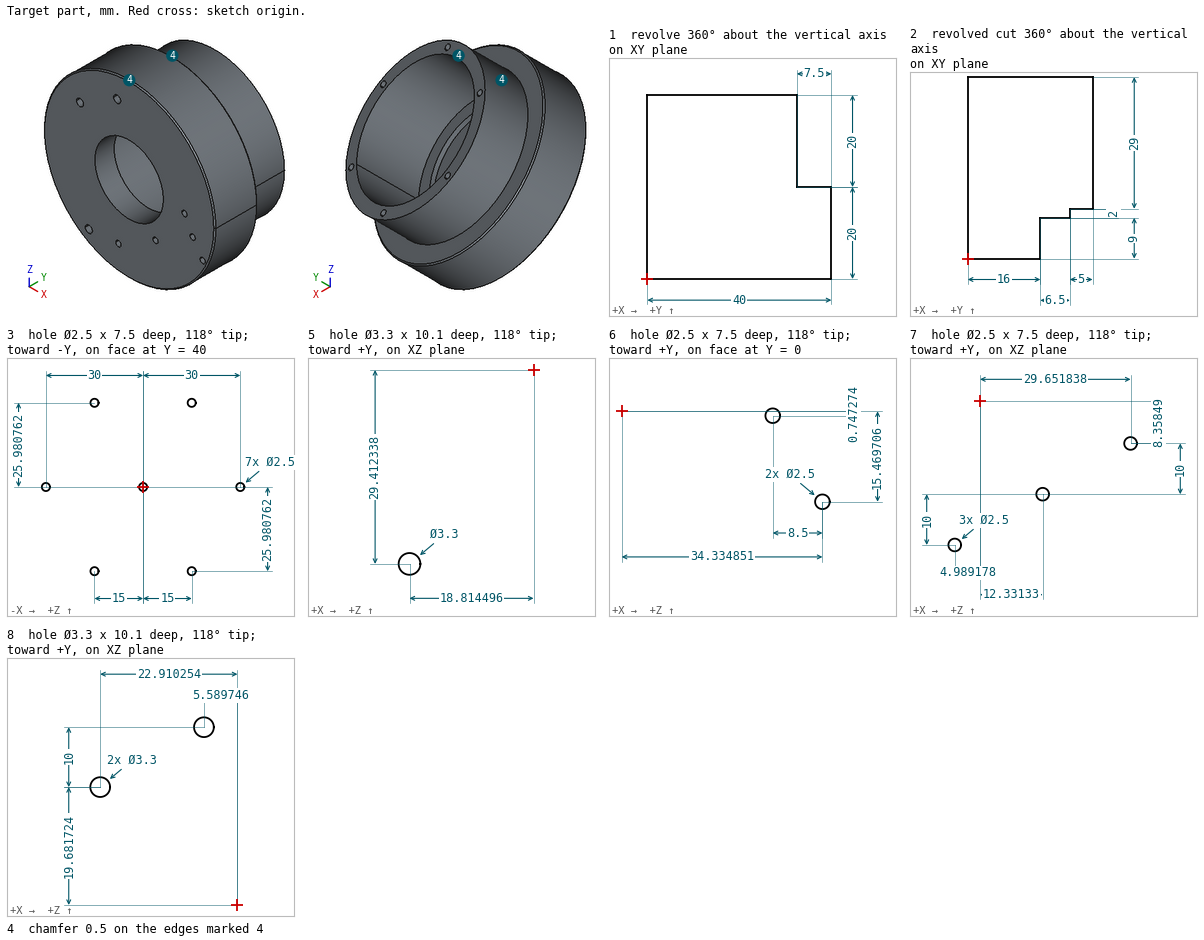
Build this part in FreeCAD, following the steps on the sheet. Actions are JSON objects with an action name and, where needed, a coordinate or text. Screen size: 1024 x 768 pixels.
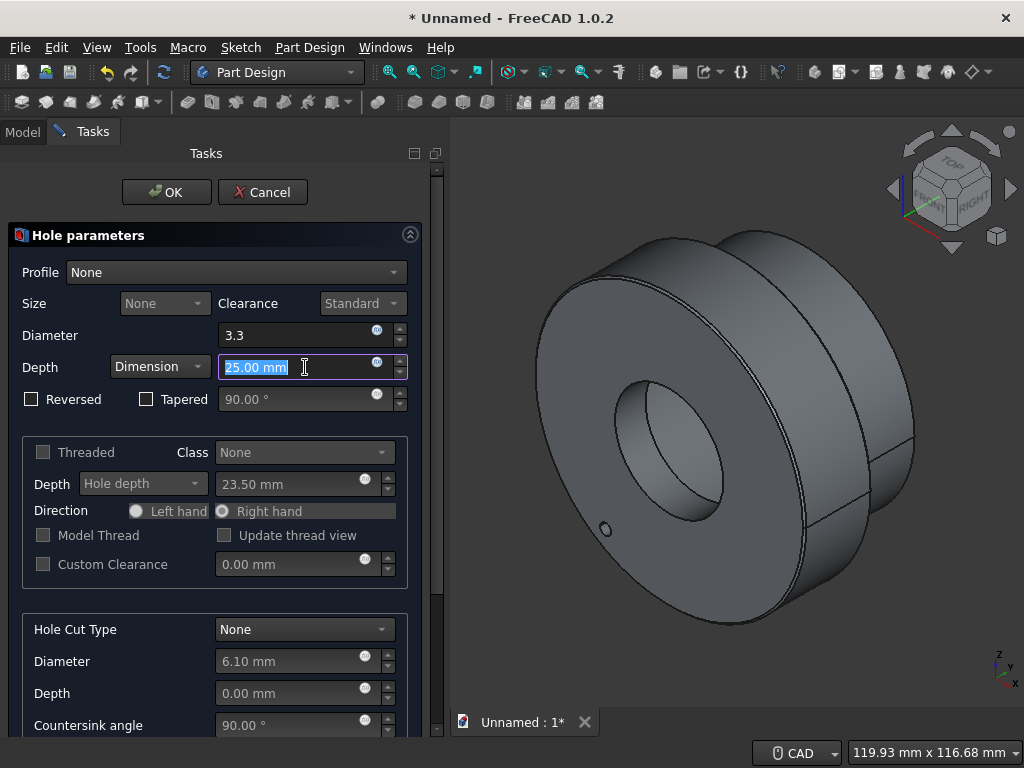
{"action": "type", "text": "10.1"}
{"action": "key", "text": "Tab"}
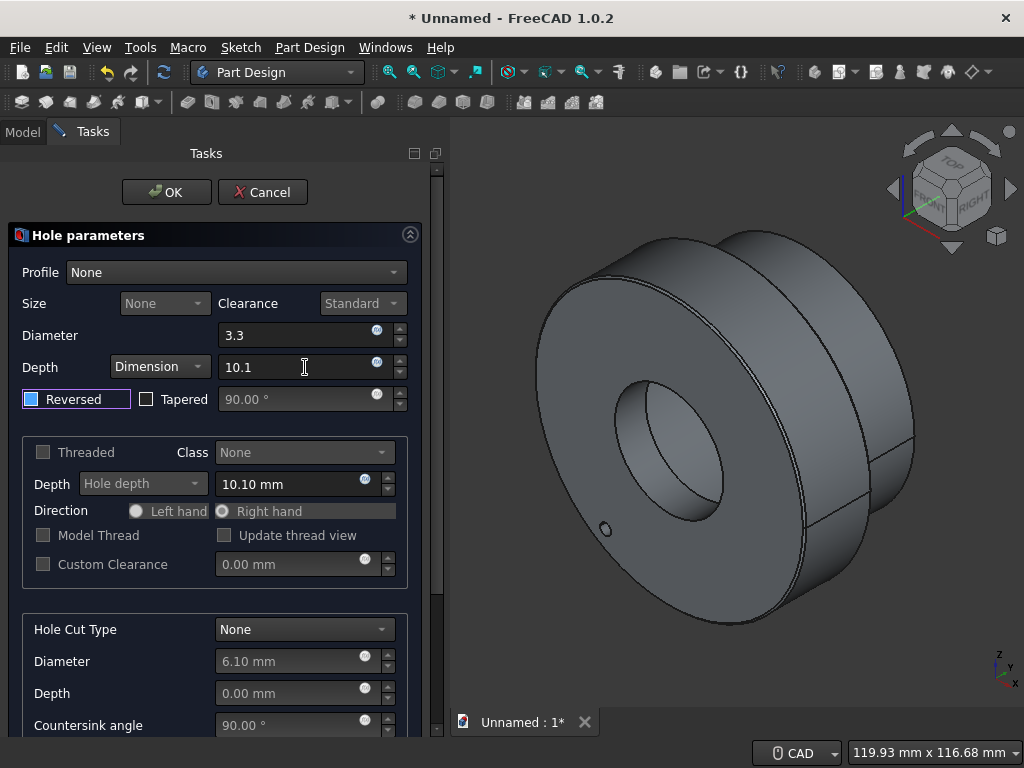
{"action": "left_click", "coordinate": [167, 192]}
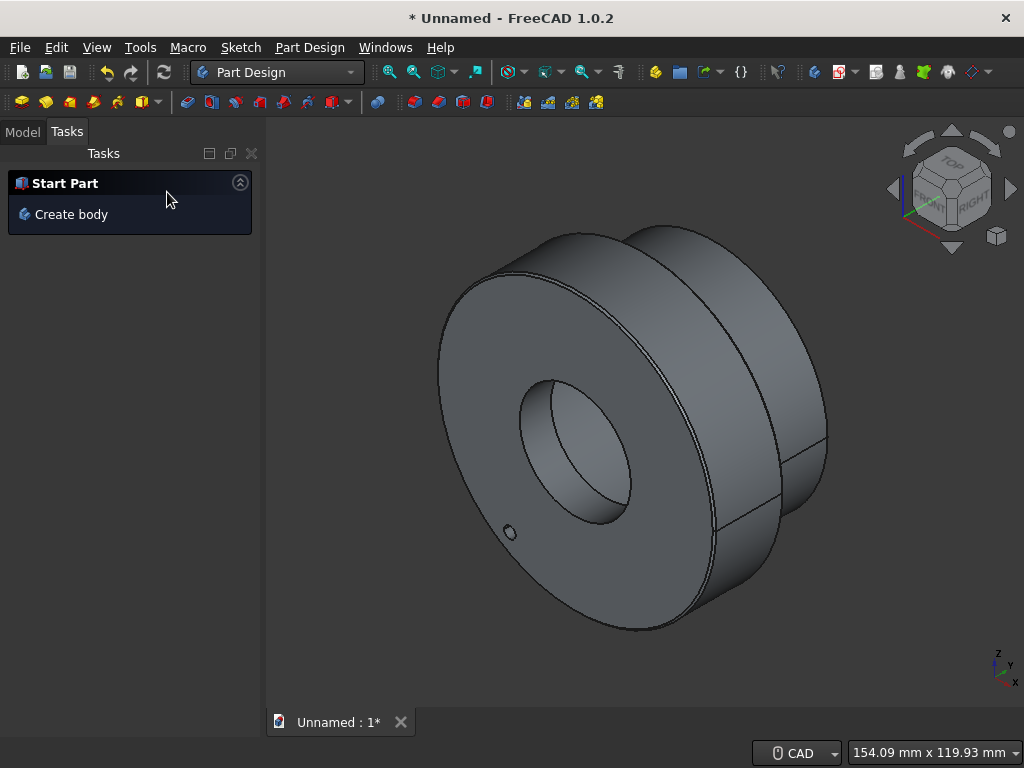
{"action": "left_click", "coordinate": [654, 451]}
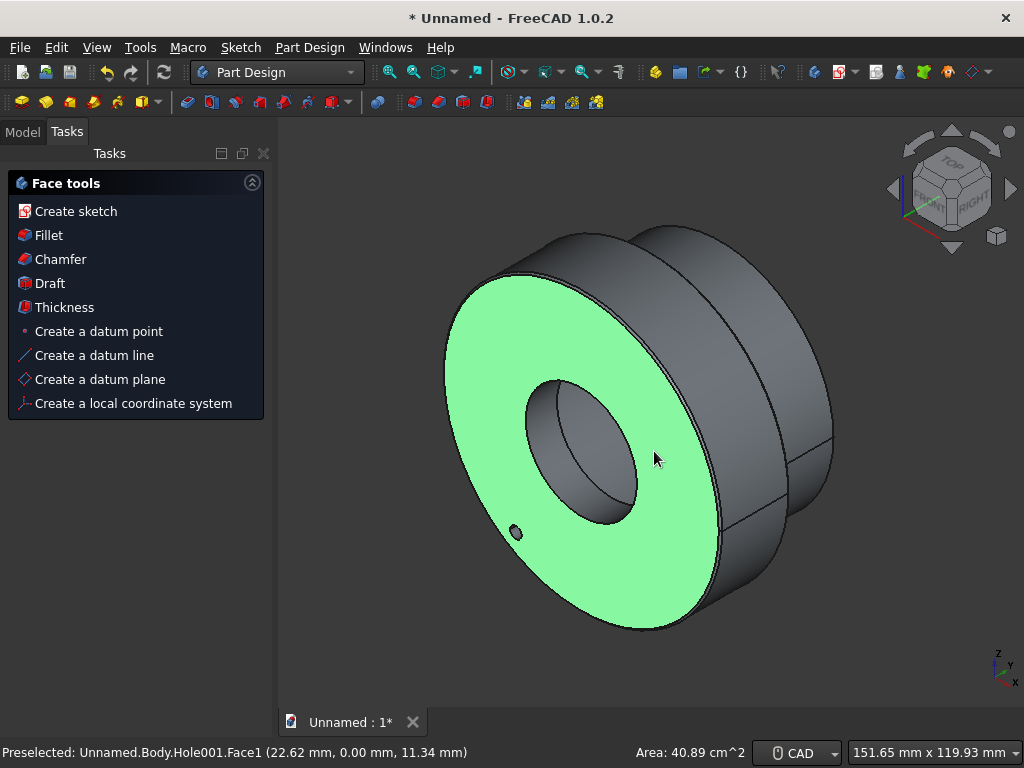
{"action": "left_click", "coordinate": [840, 72]}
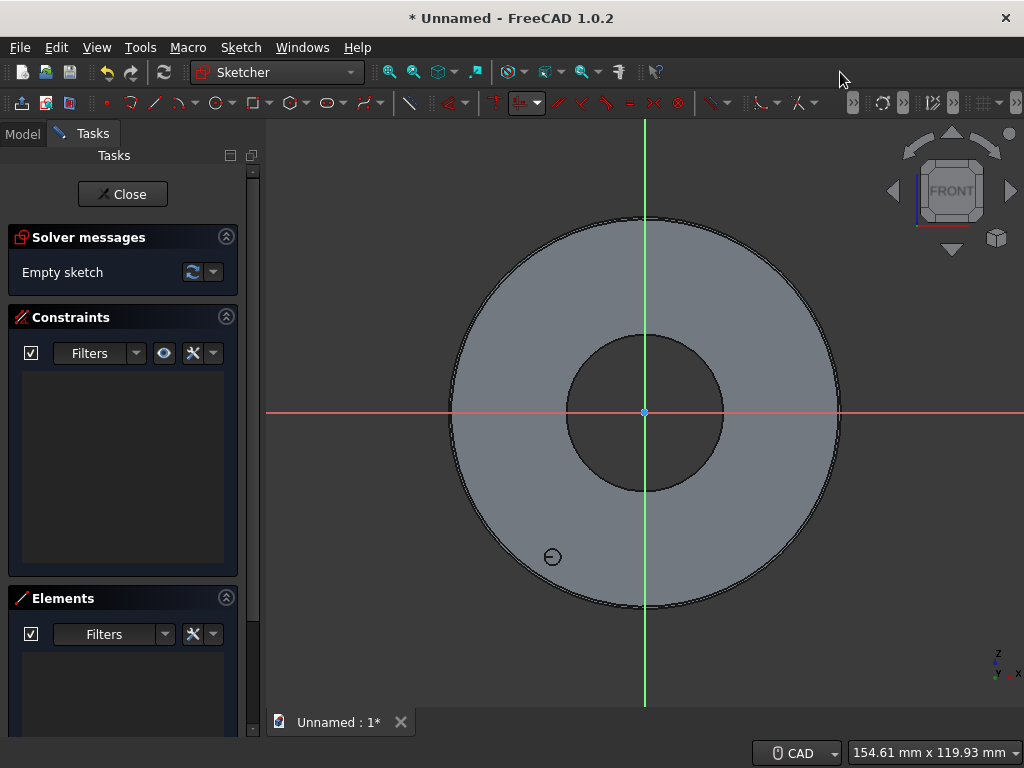
{"action": "scroll", "coordinate": [859, 485], "scroll_direction": "up", "scroll_amount": 4}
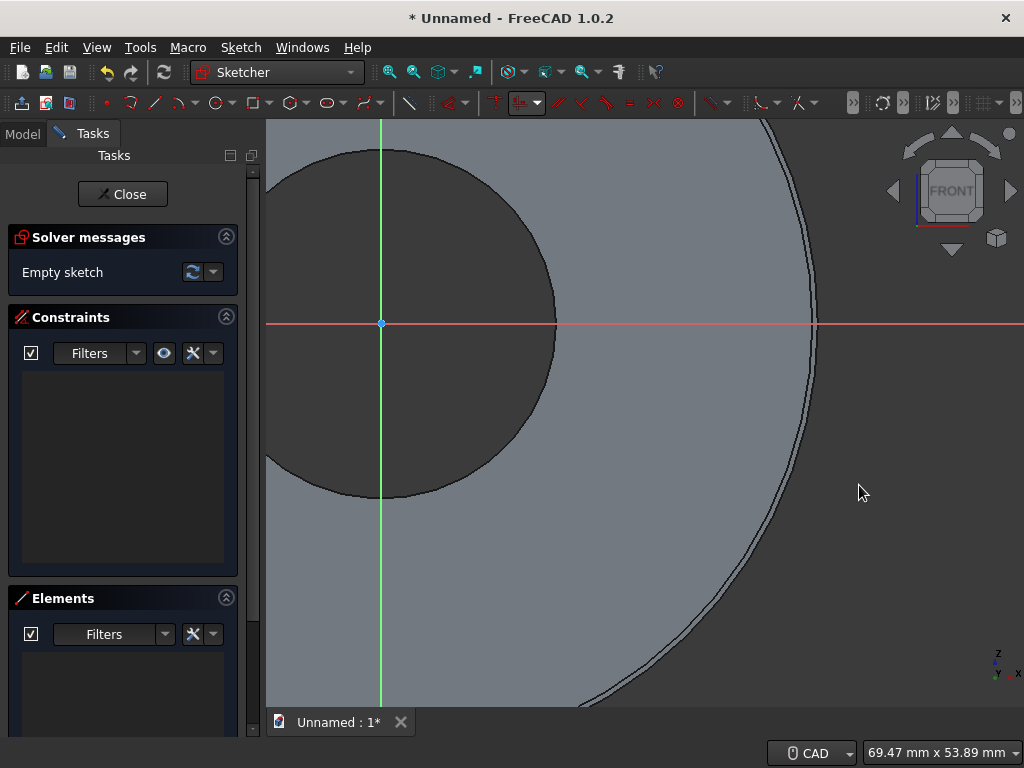
{"action": "left_click", "coordinate": [216, 104]}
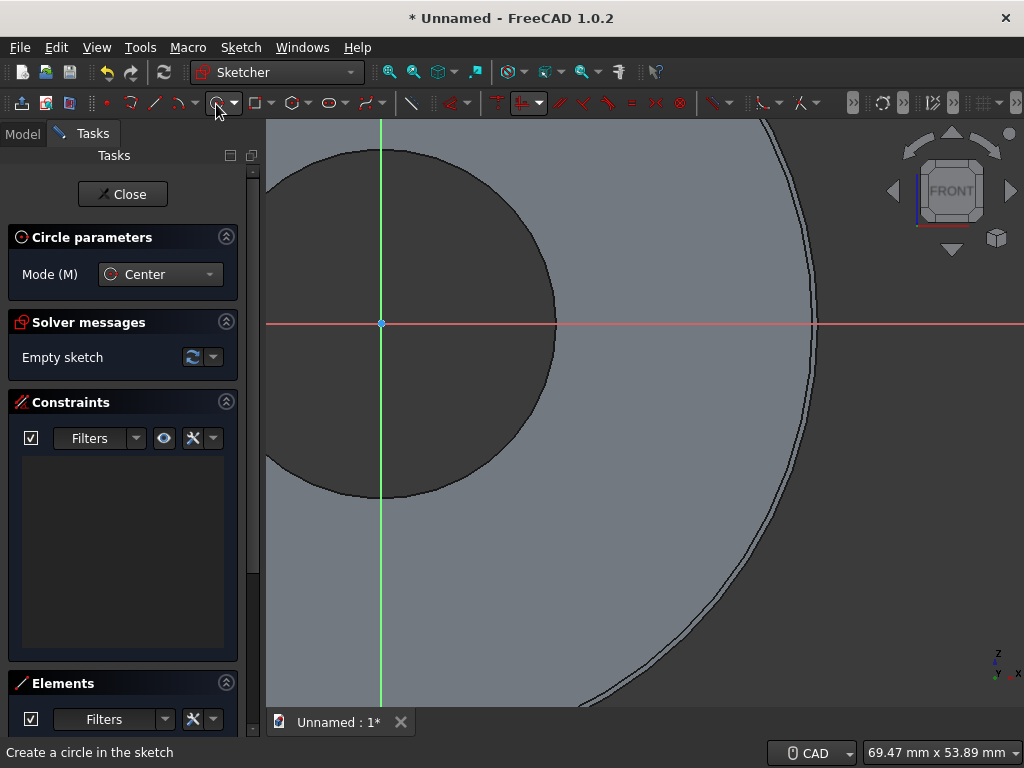
{"action": "scroll", "coordinate": [756, 493], "scroll_direction": "up", "scroll_amount": 3}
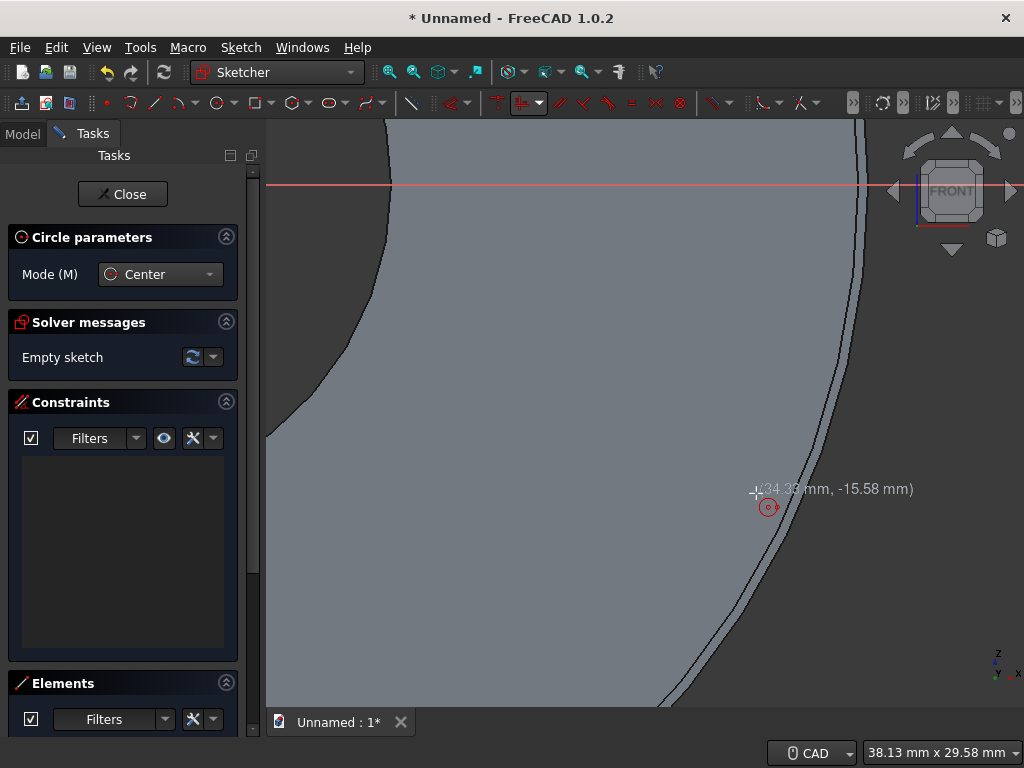
{"action": "left_click", "coordinate": [756, 492]}
{"action": "mouse_move", "coordinate": [773, 475]}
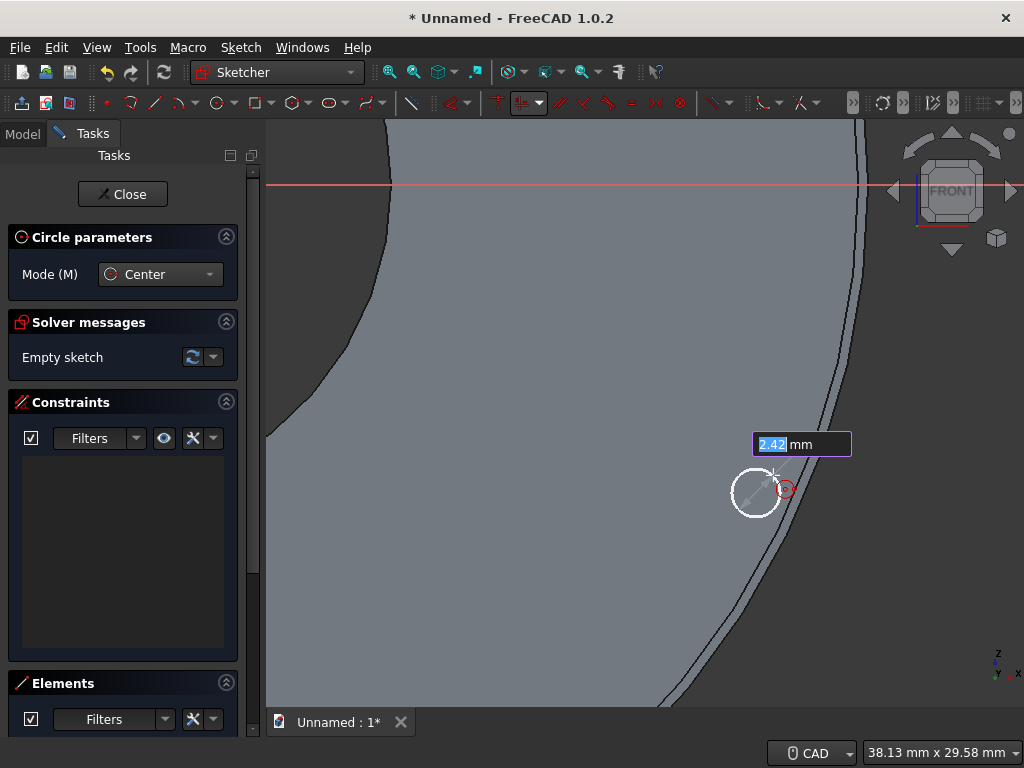
{"action": "type", "text": "2.5"}
{"action": "key", "text": "Return"}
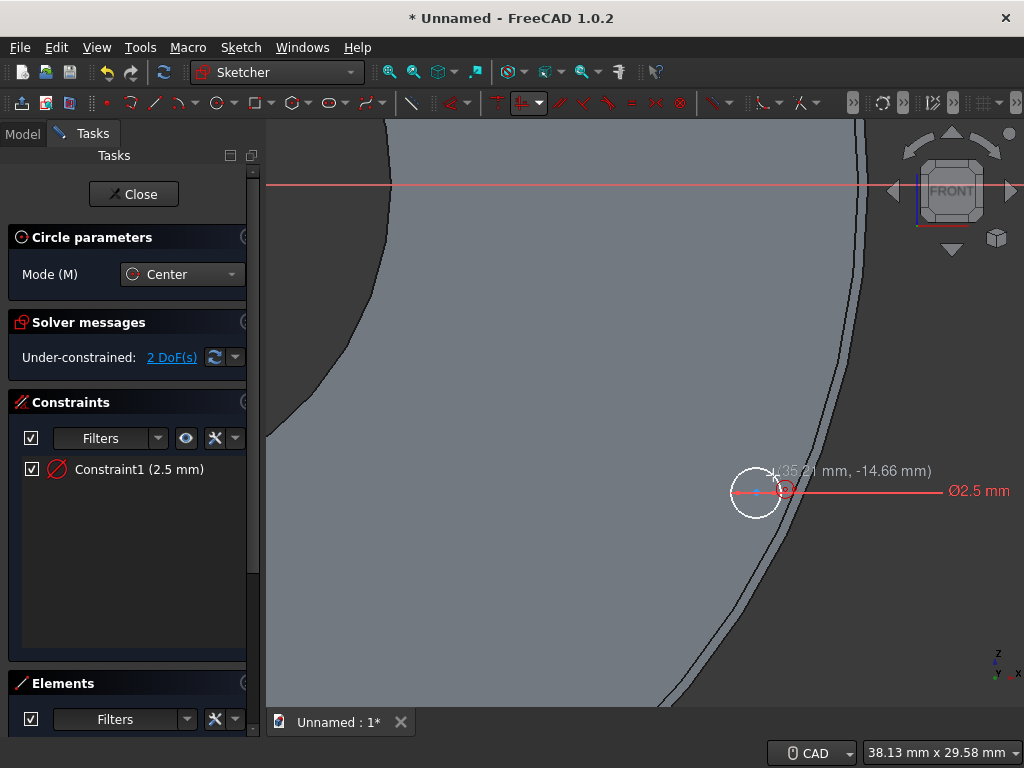
{"action": "left_click", "coordinate": [587, 199]}
{"action": "mouse_move", "coordinate": [604, 217]}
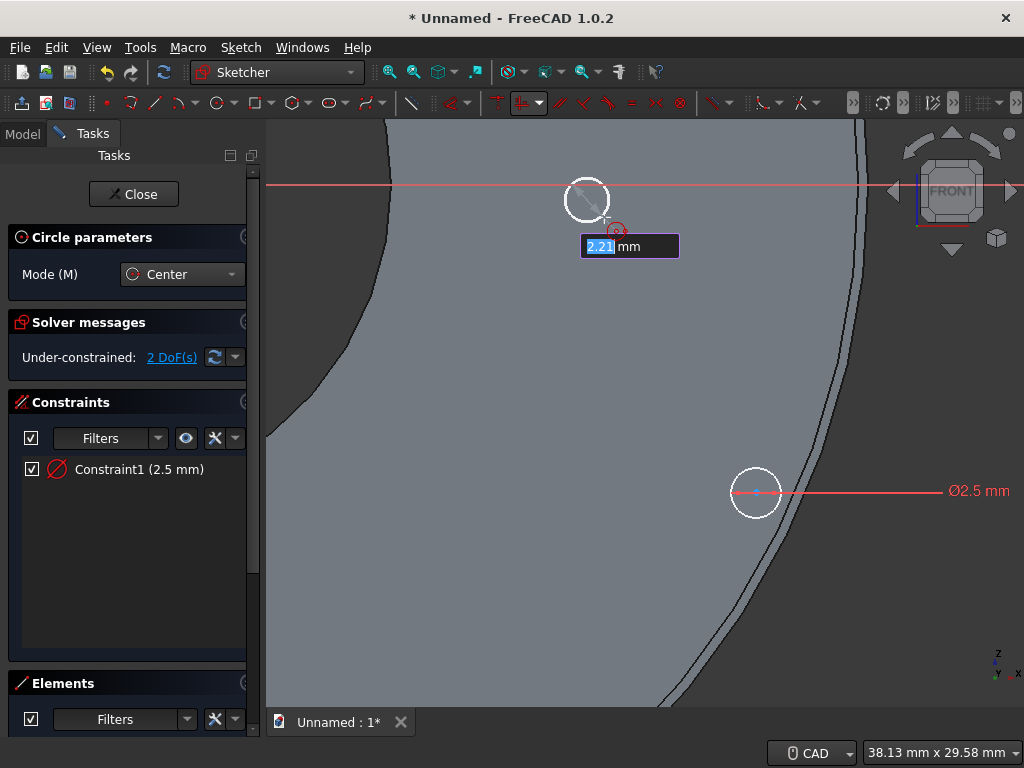
{"action": "type", "text": "2.5"}
{"action": "key", "text": "Return"}
{"action": "key", "text": "Escape"}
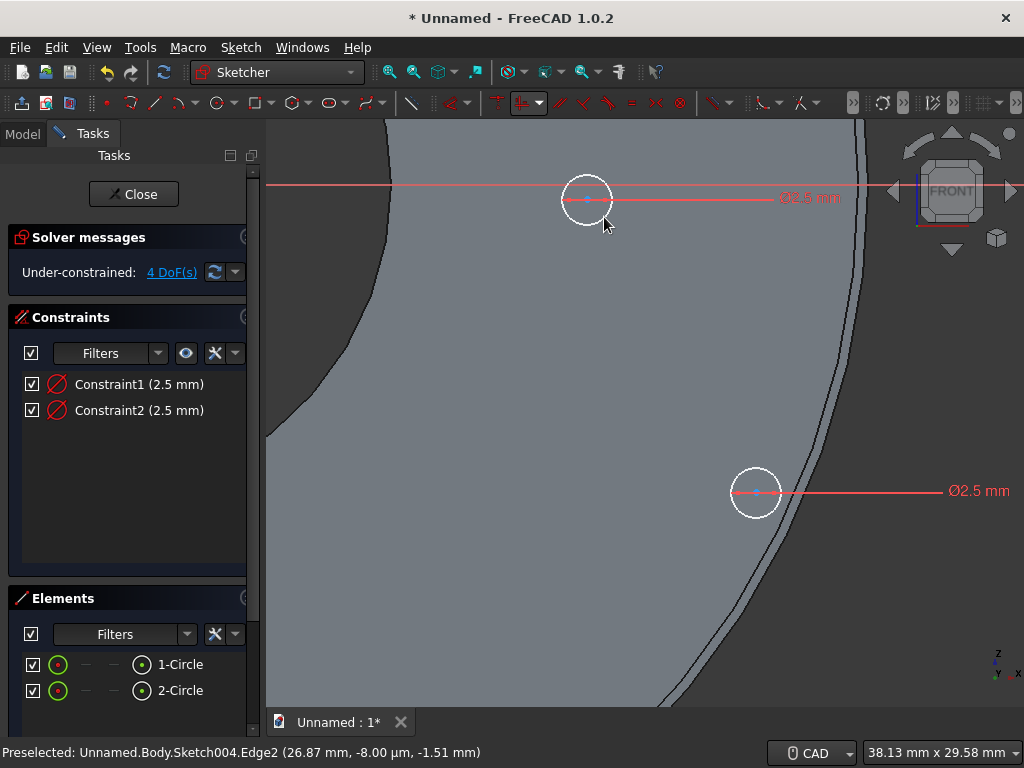
{"action": "left_click", "coordinate": [450, 104]}